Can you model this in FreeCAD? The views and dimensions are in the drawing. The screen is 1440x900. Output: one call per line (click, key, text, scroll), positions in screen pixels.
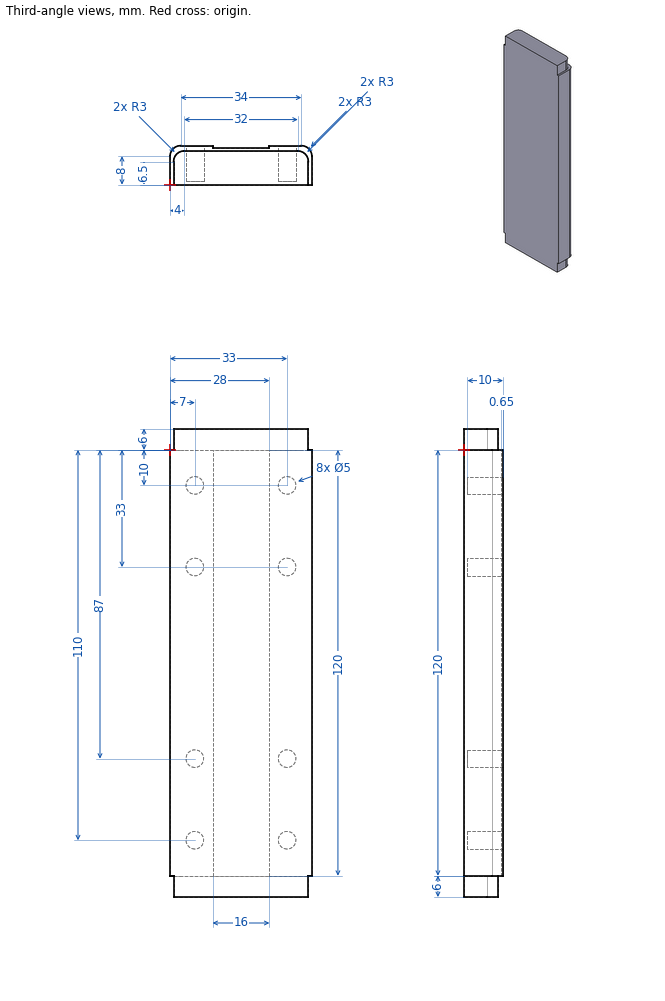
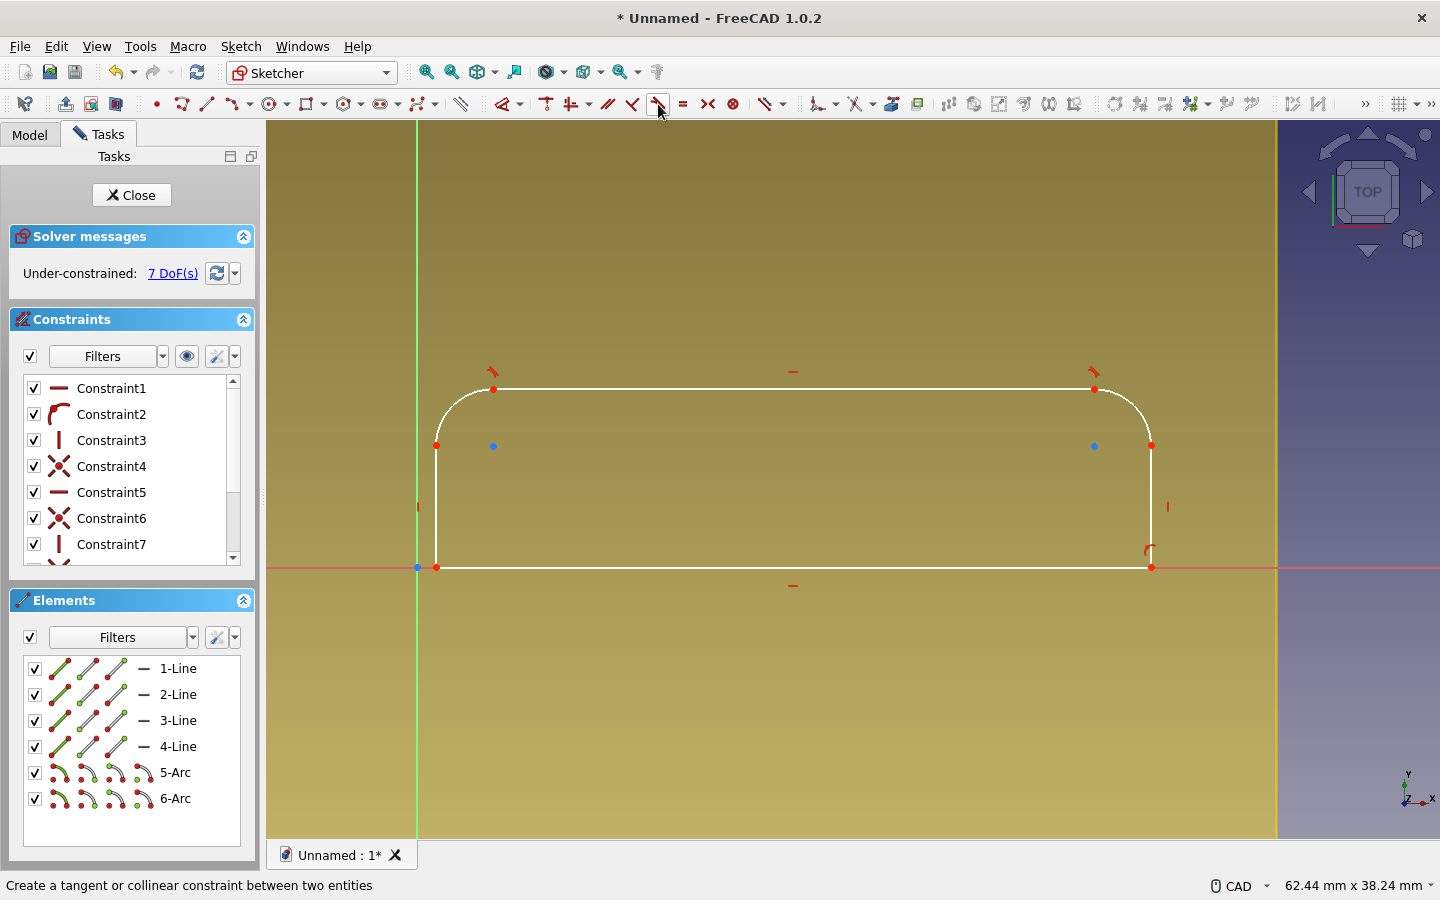
click(1151, 482)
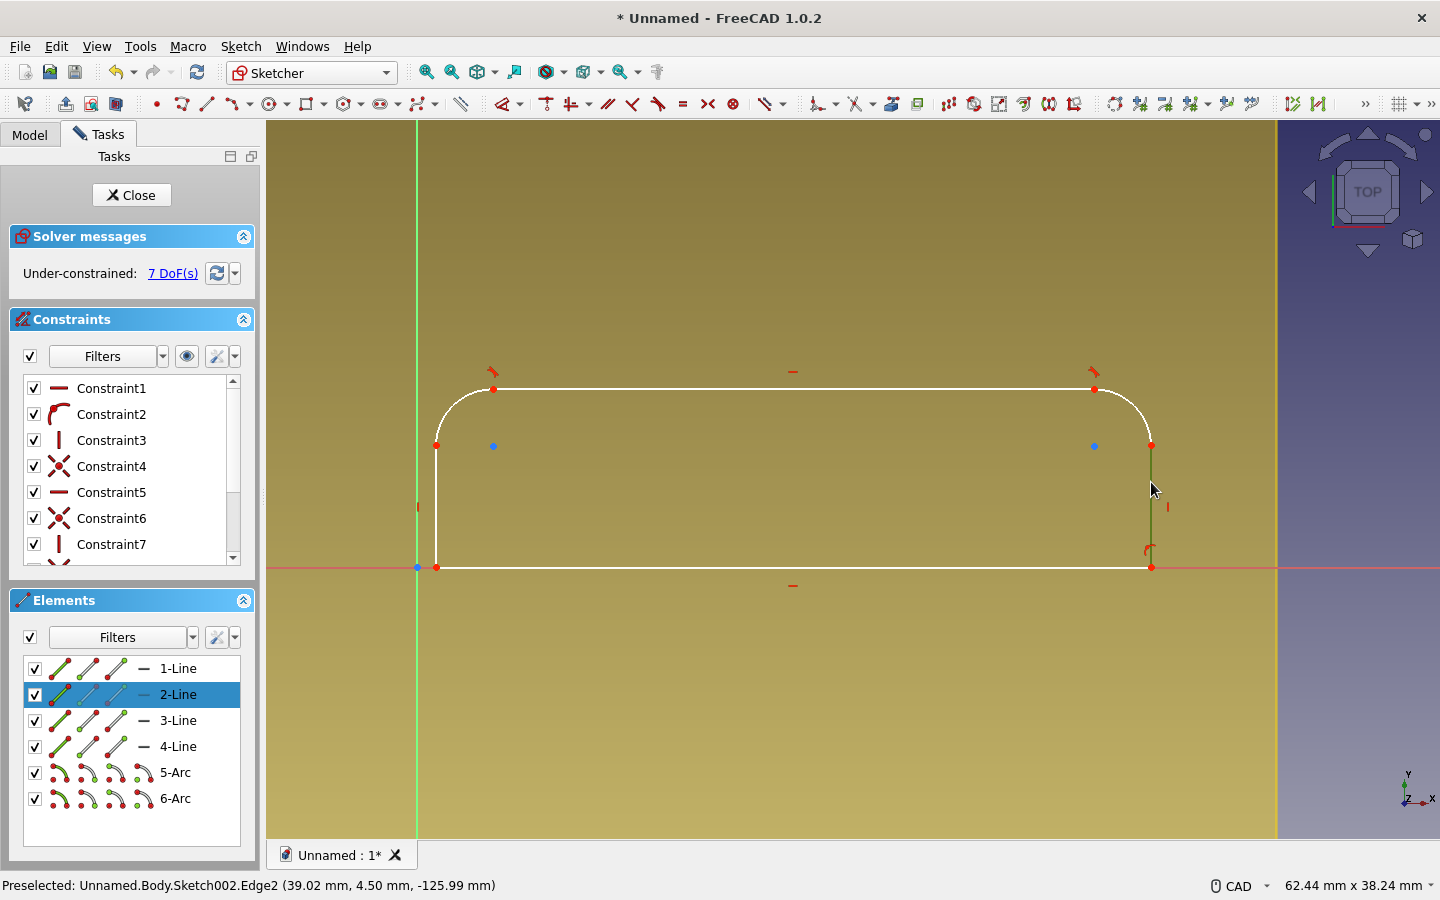
click(1145, 420)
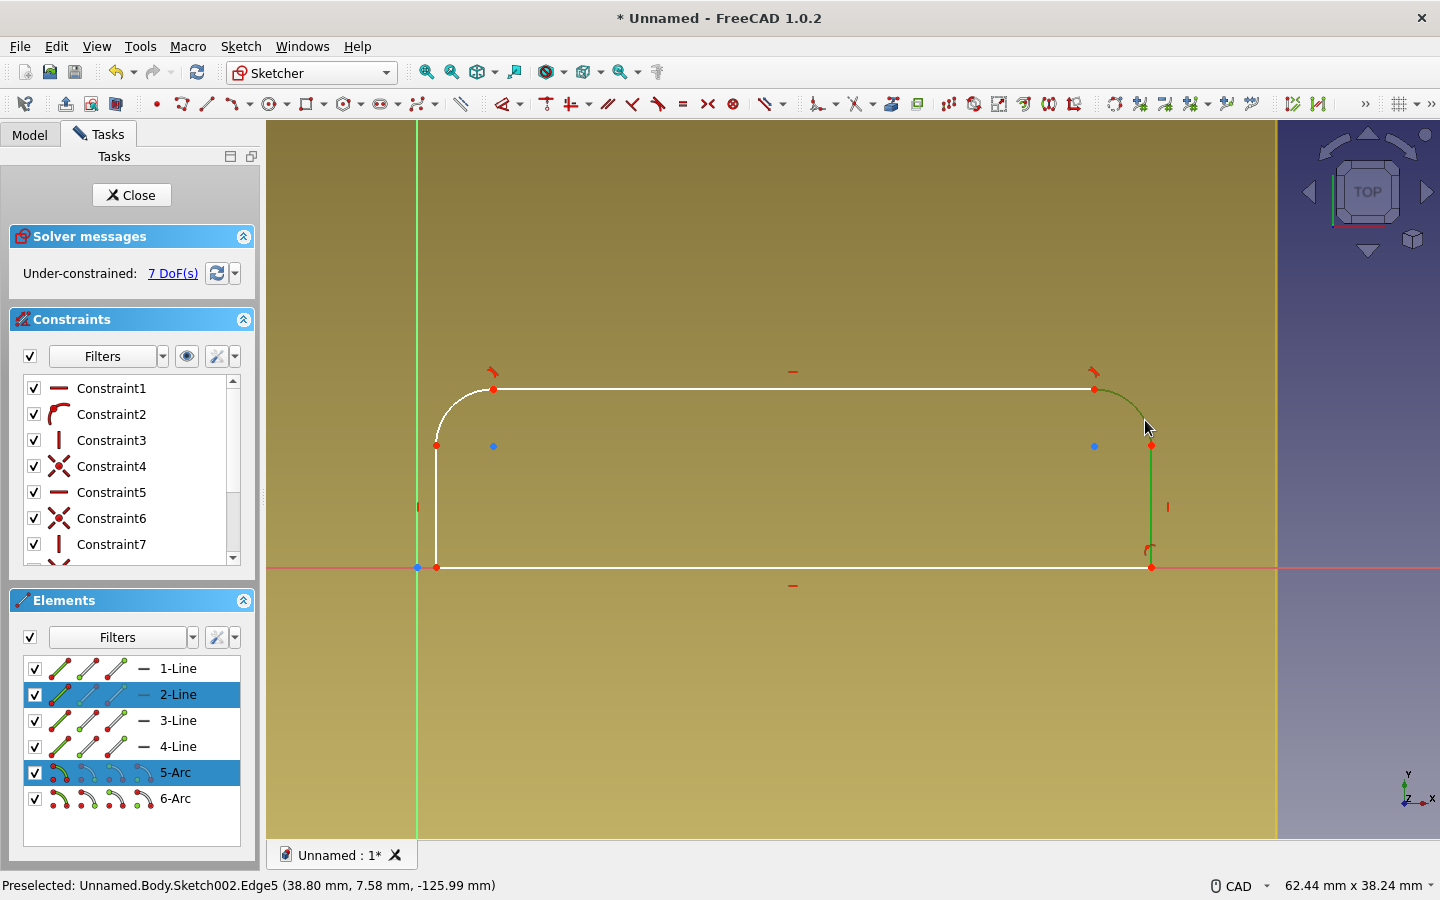
click(658, 104)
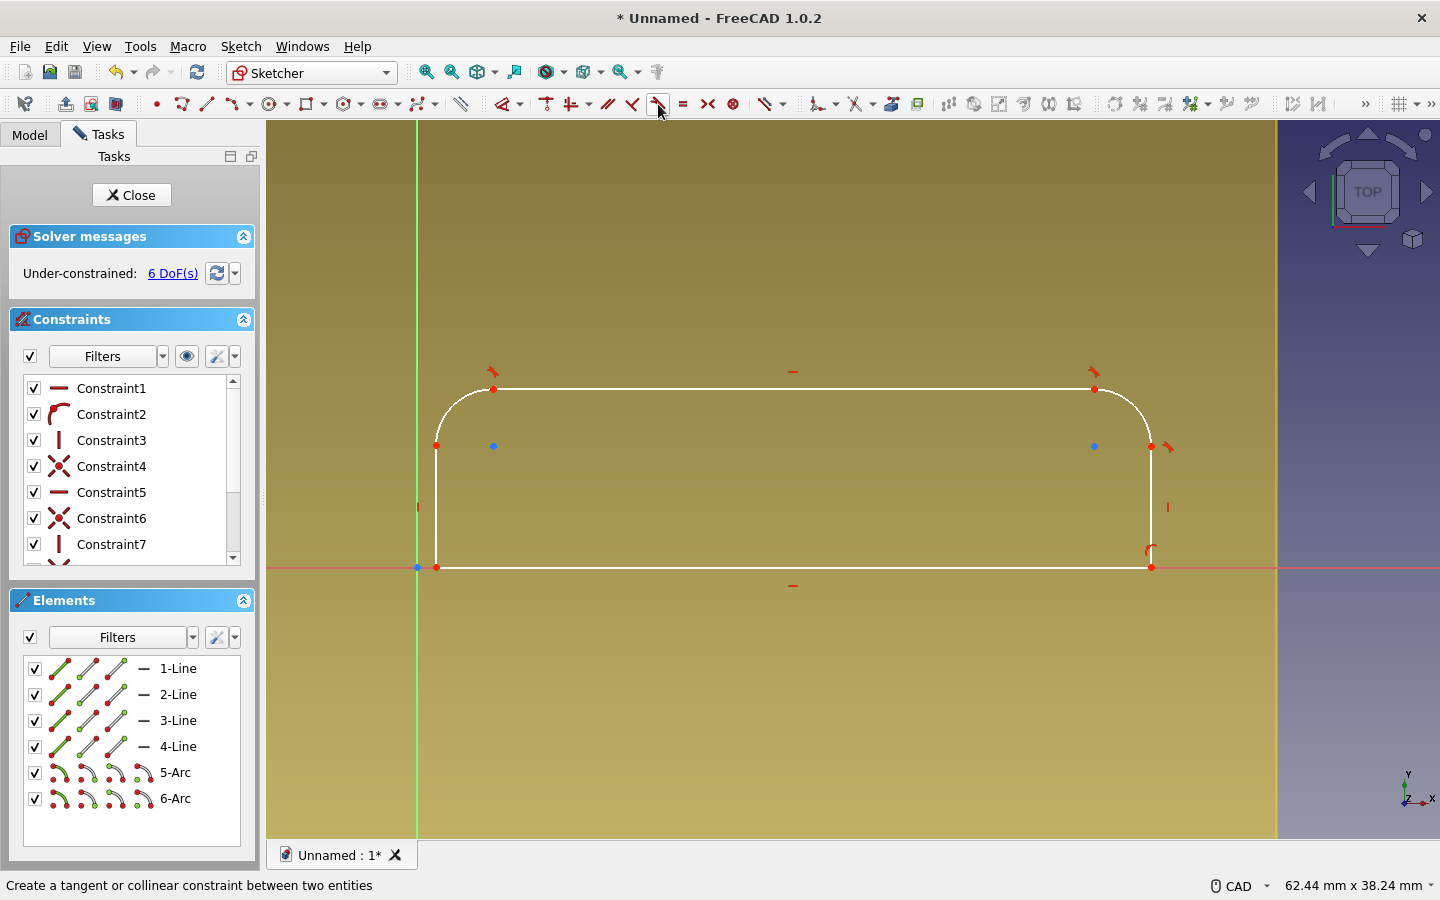
click(436, 531)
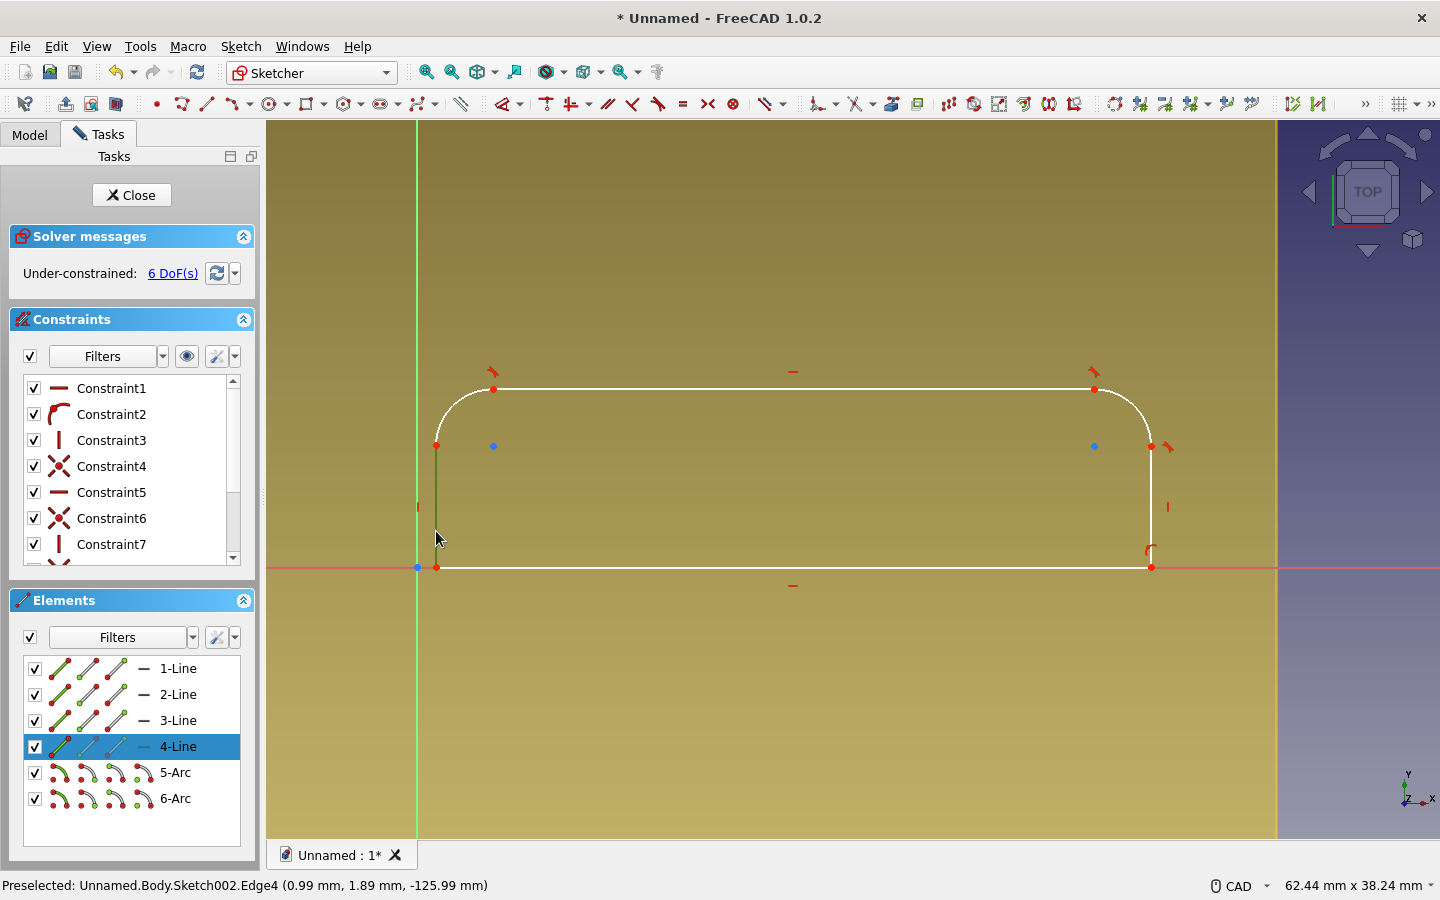
click(467, 395)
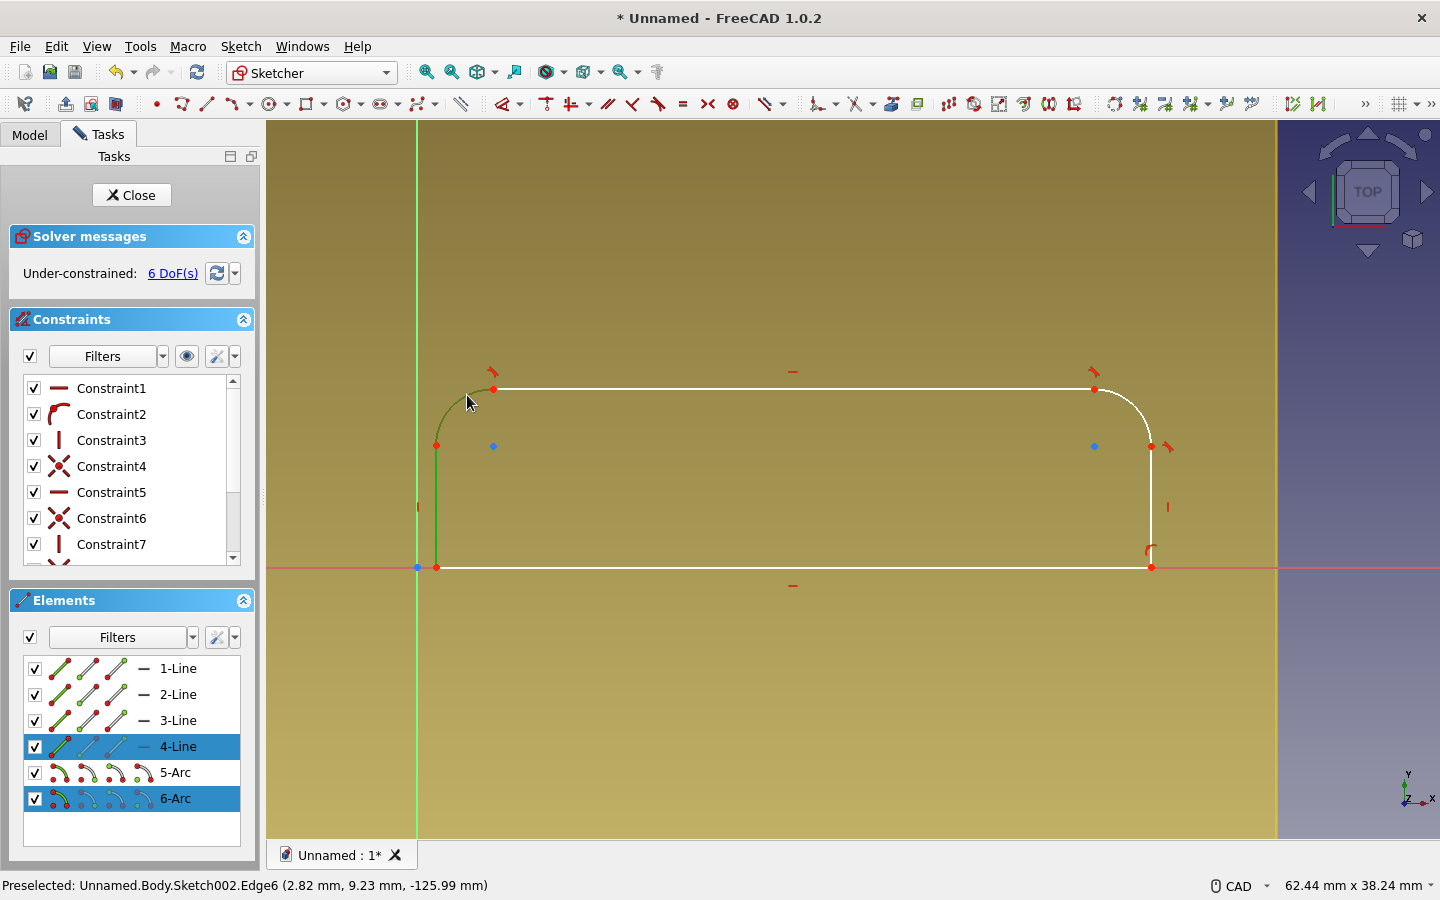
click(658, 104)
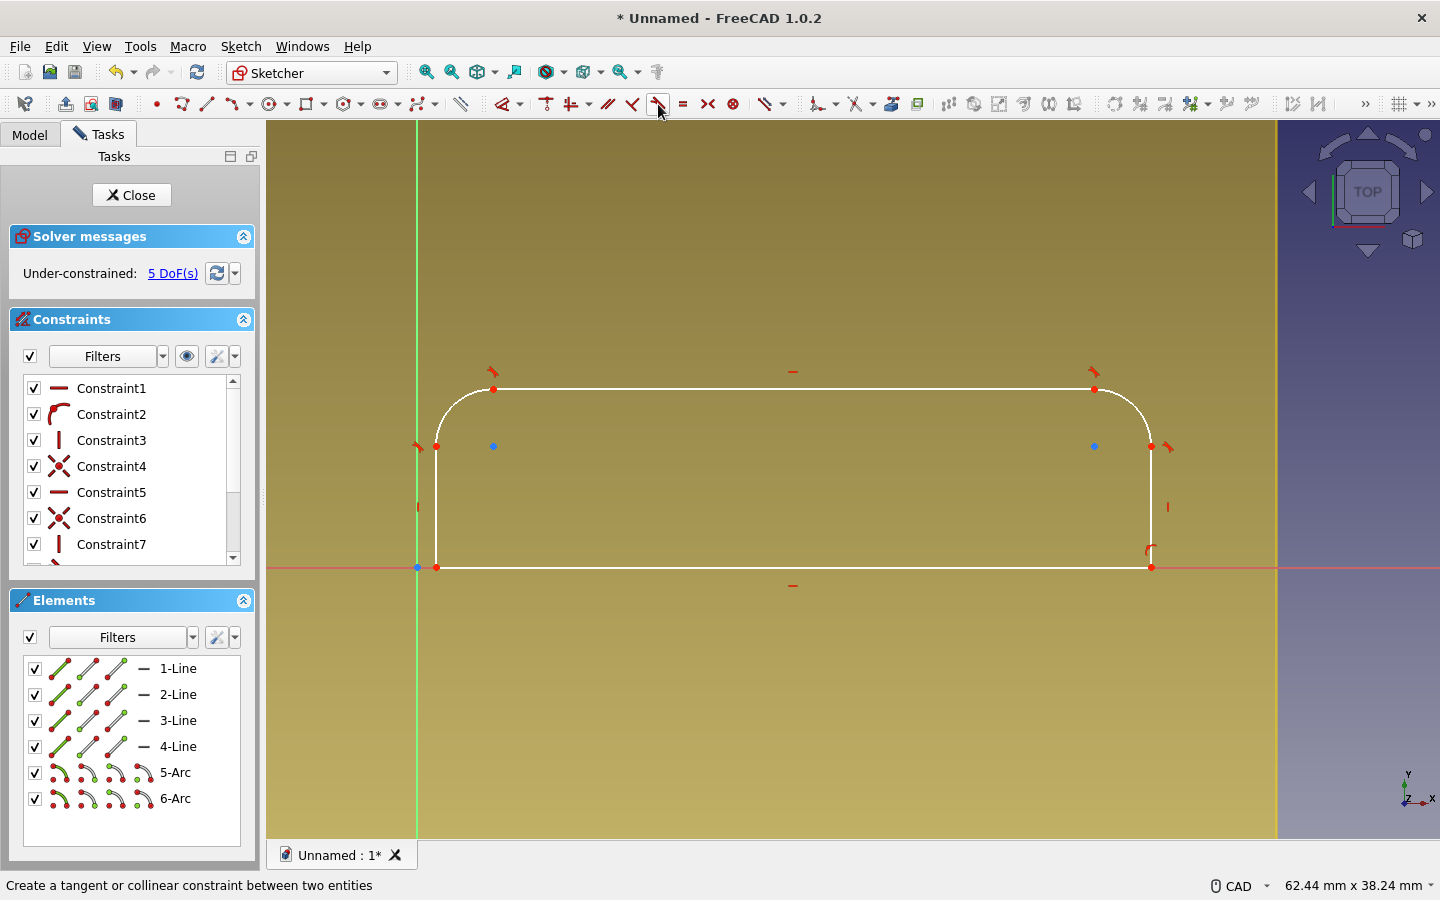
click(1145, 420)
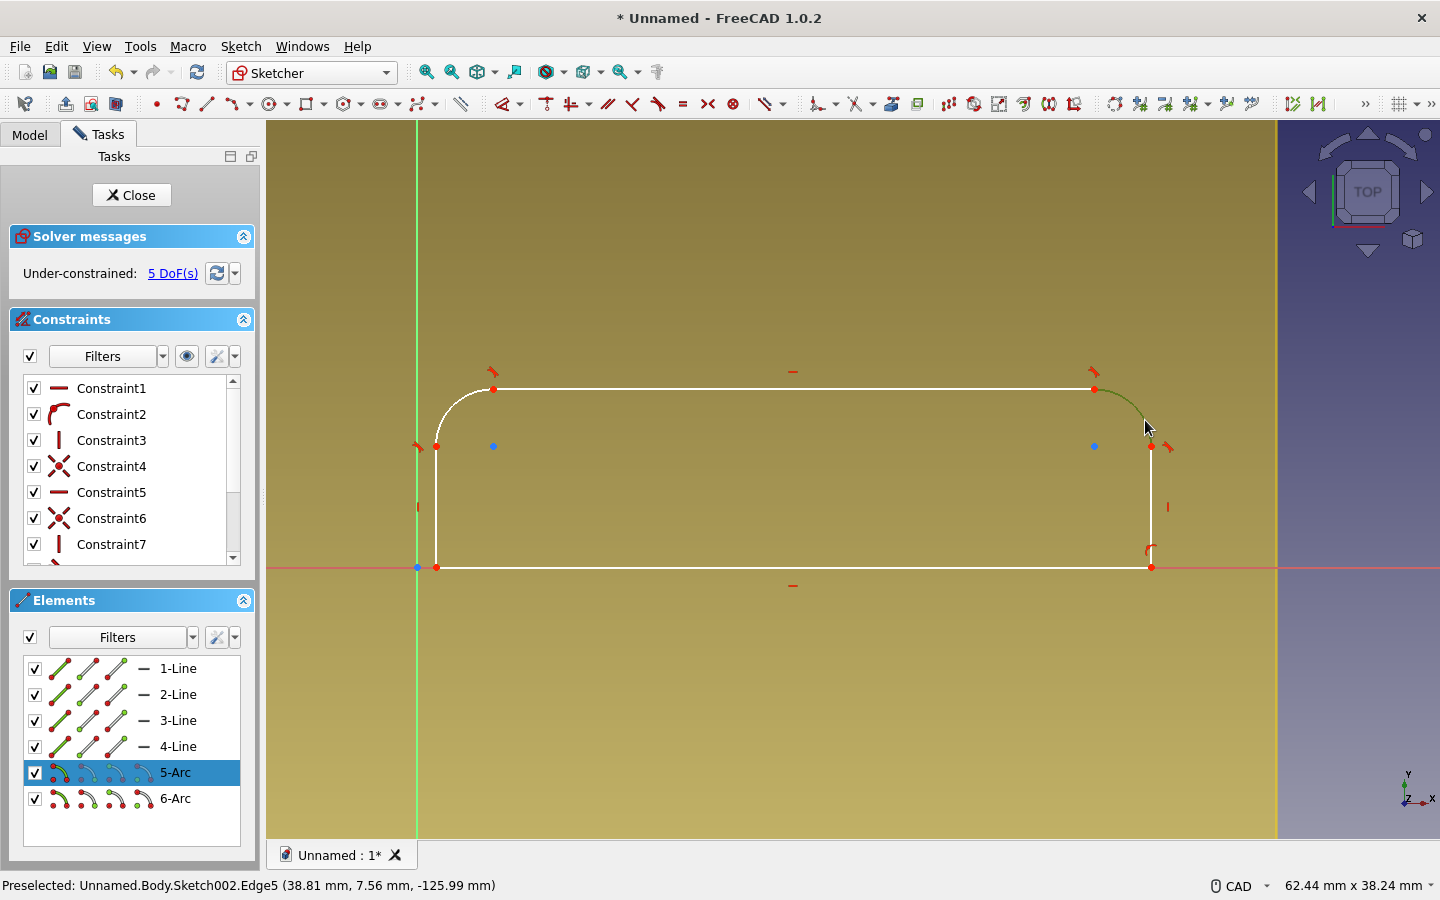
click(467, 396)